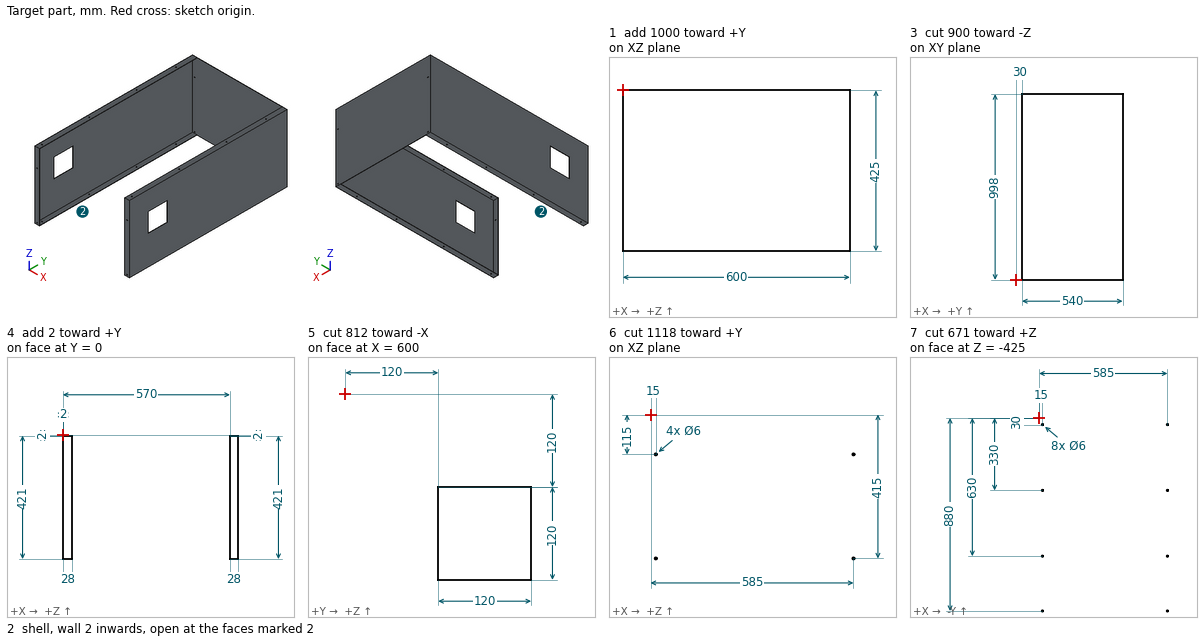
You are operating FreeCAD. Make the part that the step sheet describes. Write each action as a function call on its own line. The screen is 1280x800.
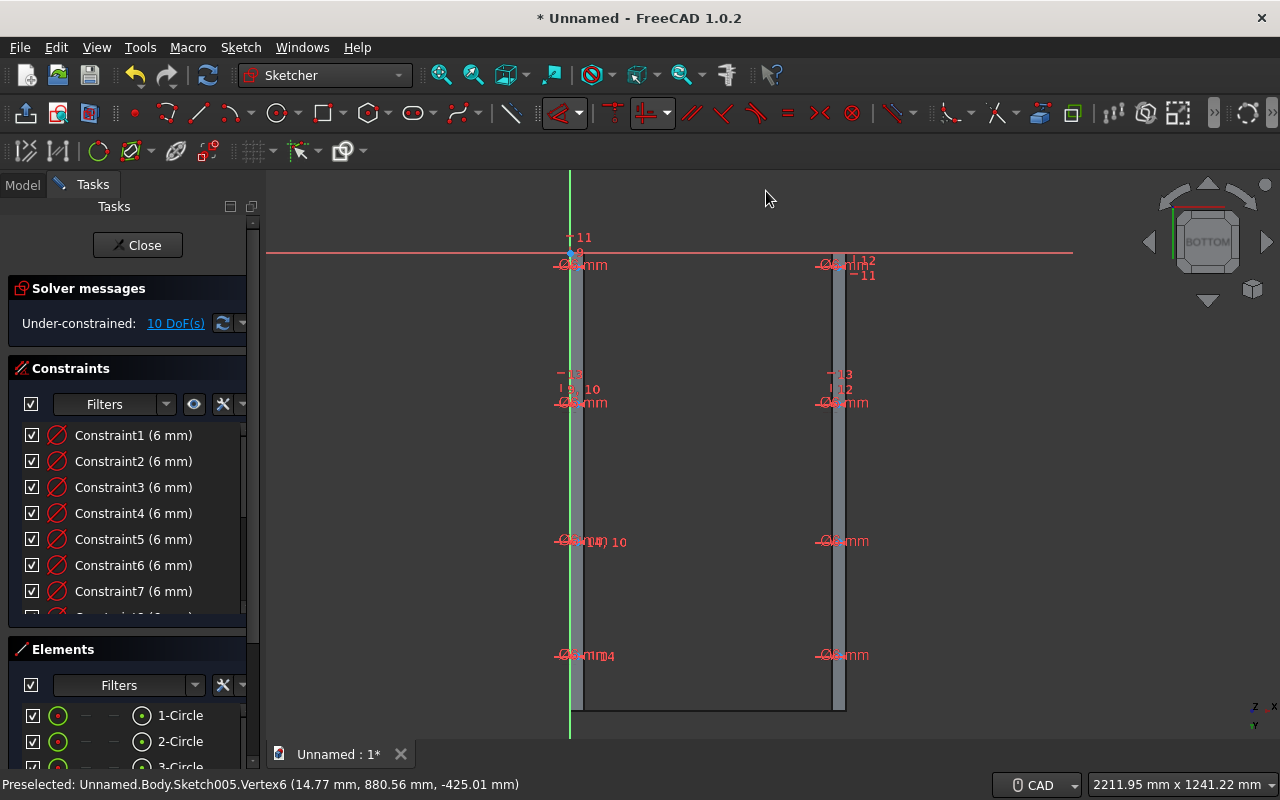
click(838, 405)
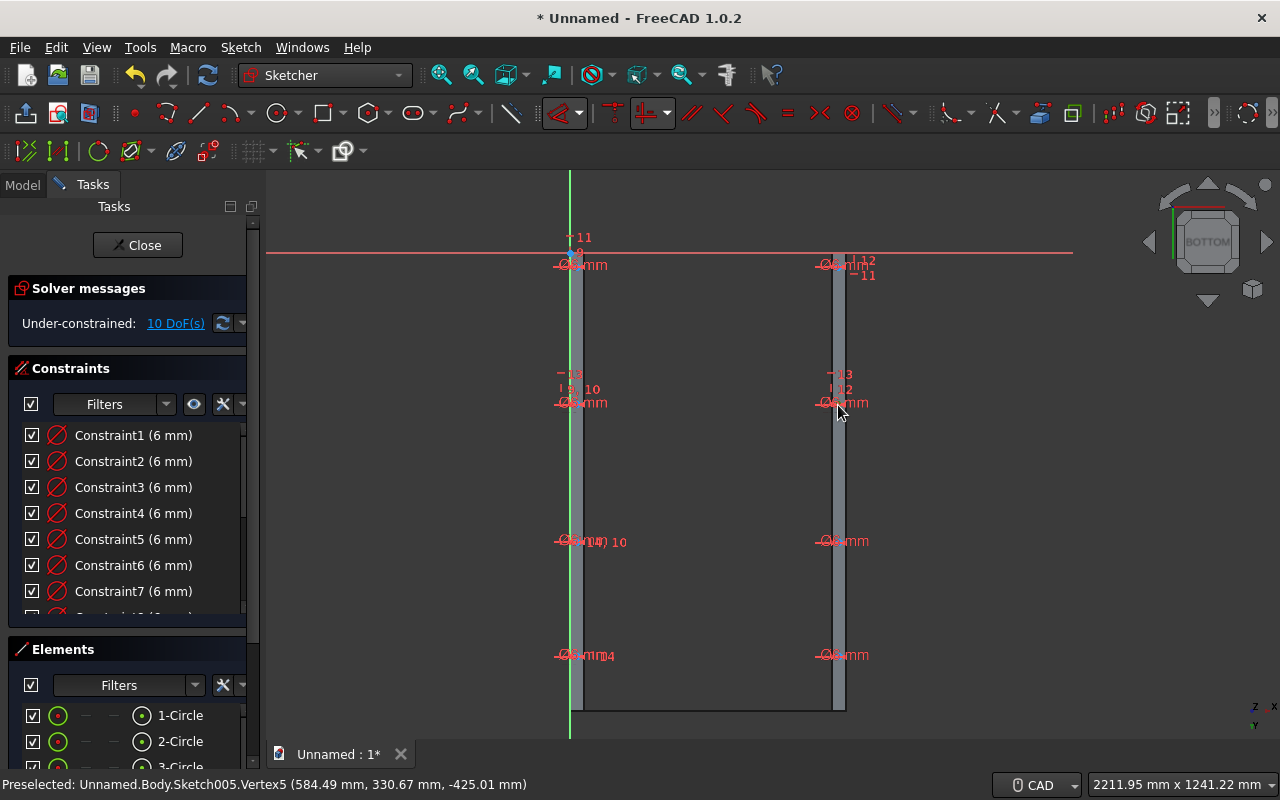
click(839, 543)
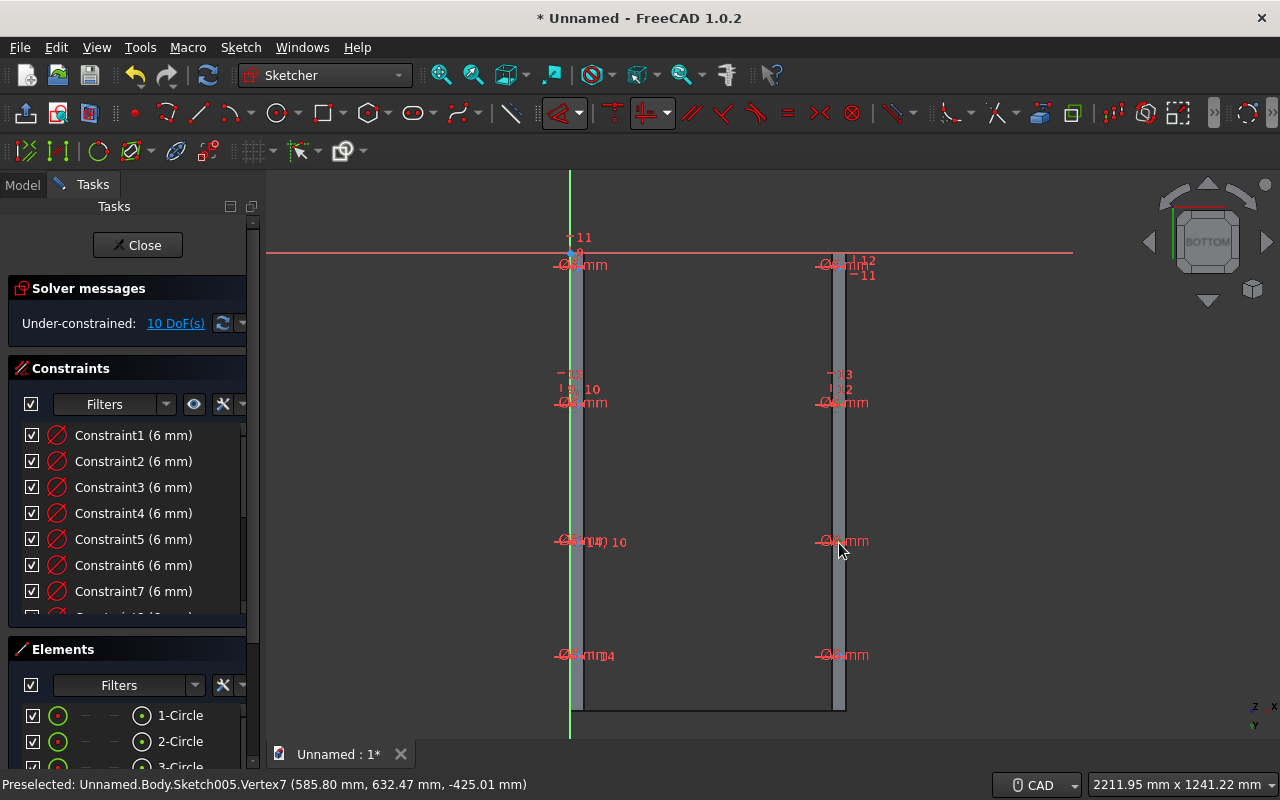
key(v)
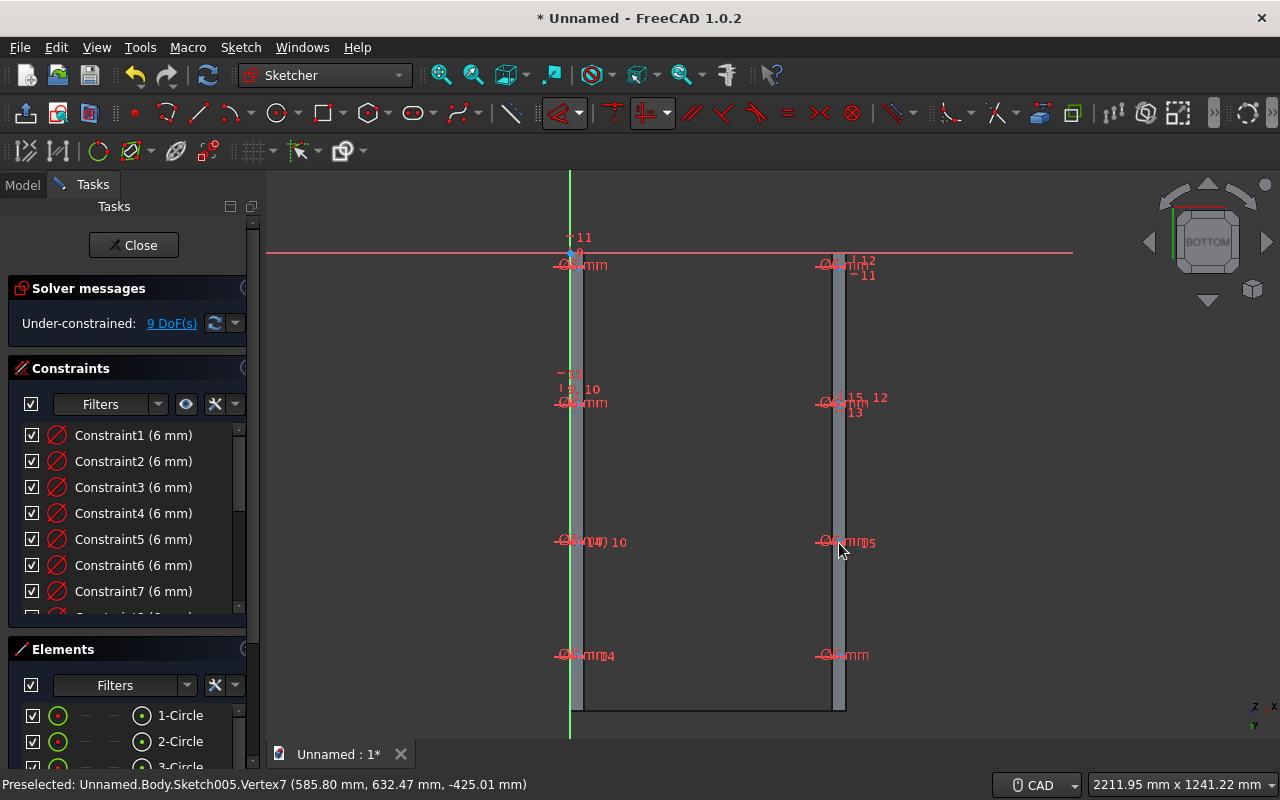
click(577, 542)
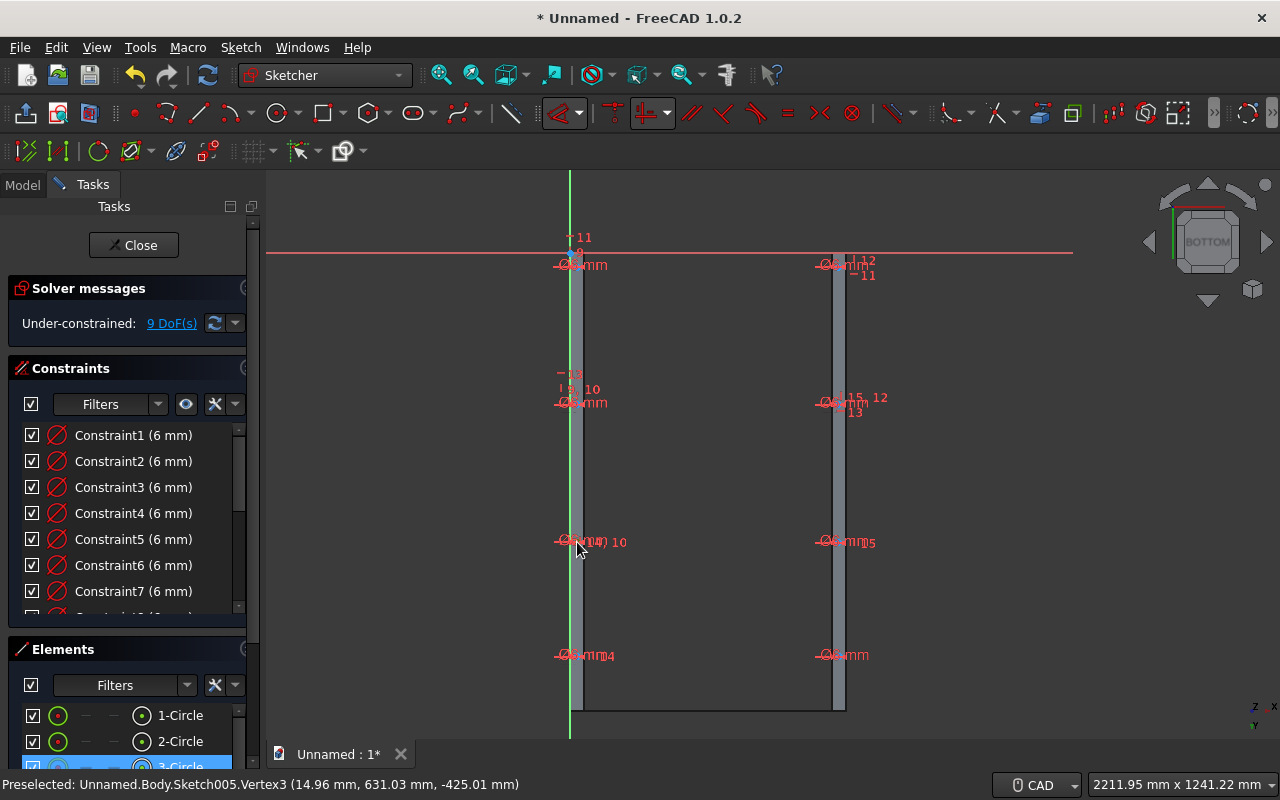
click(838, 543)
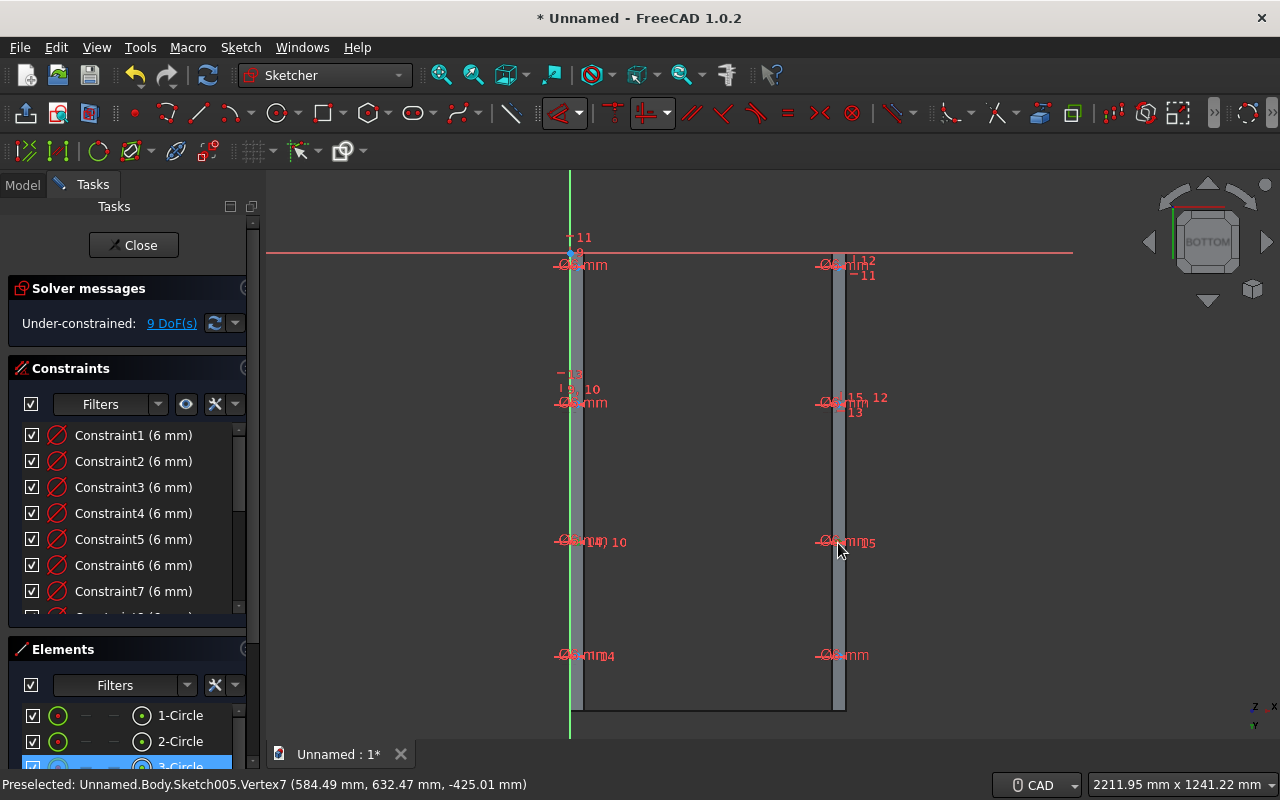
click(670, 114)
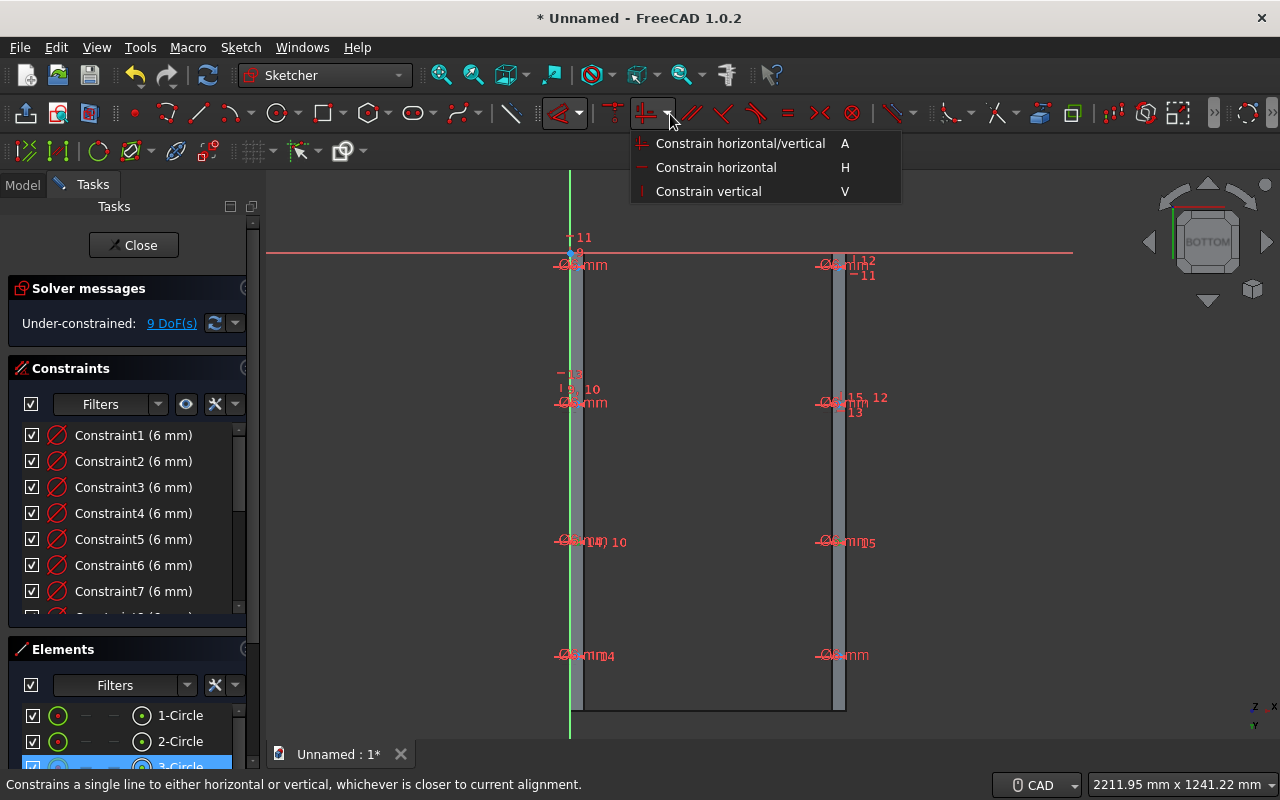
click(766, 167)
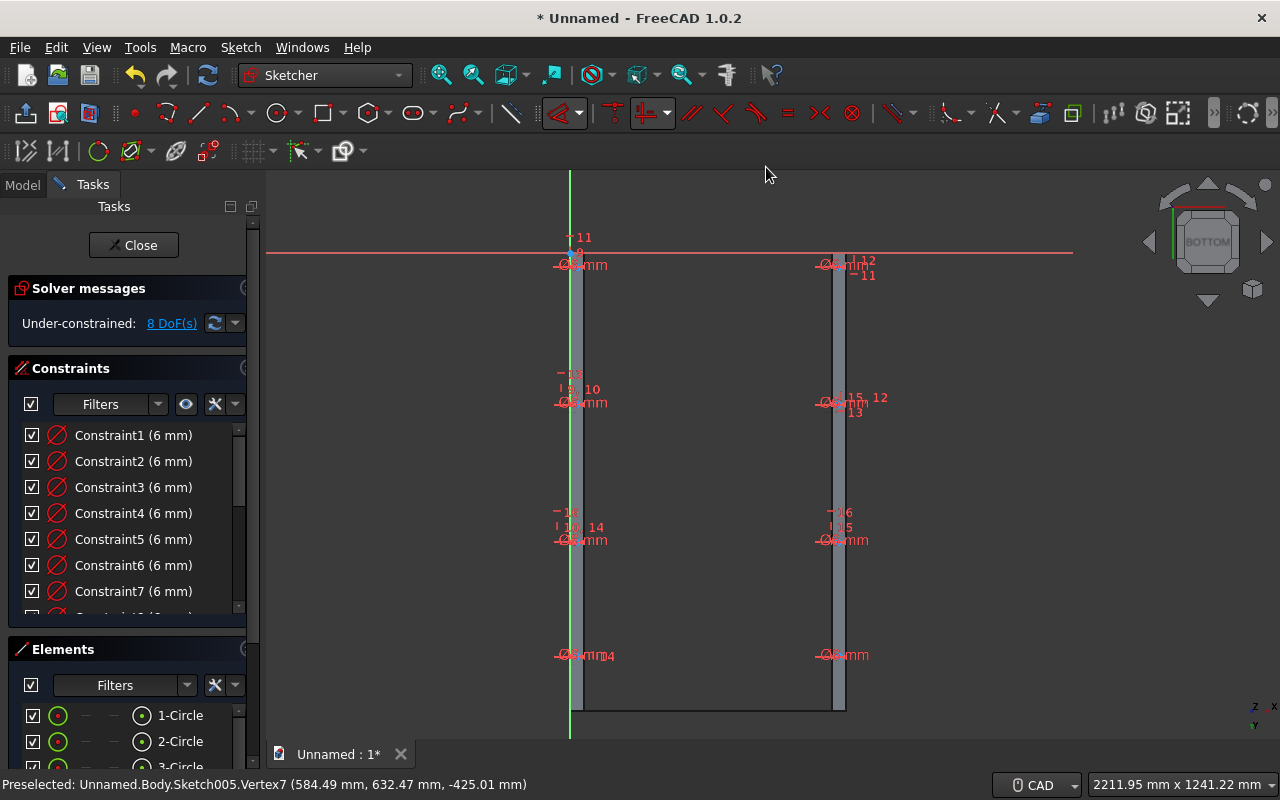
click(838, 542)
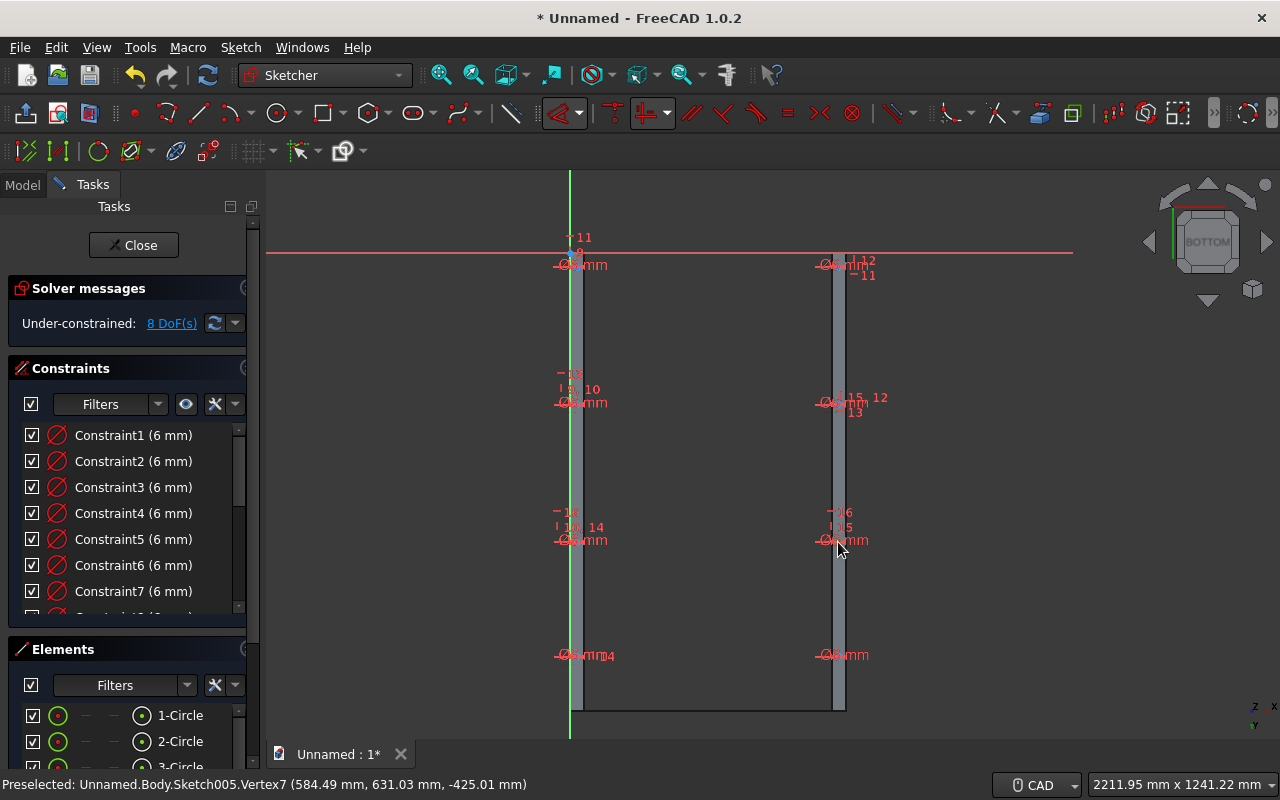
click(839, 657)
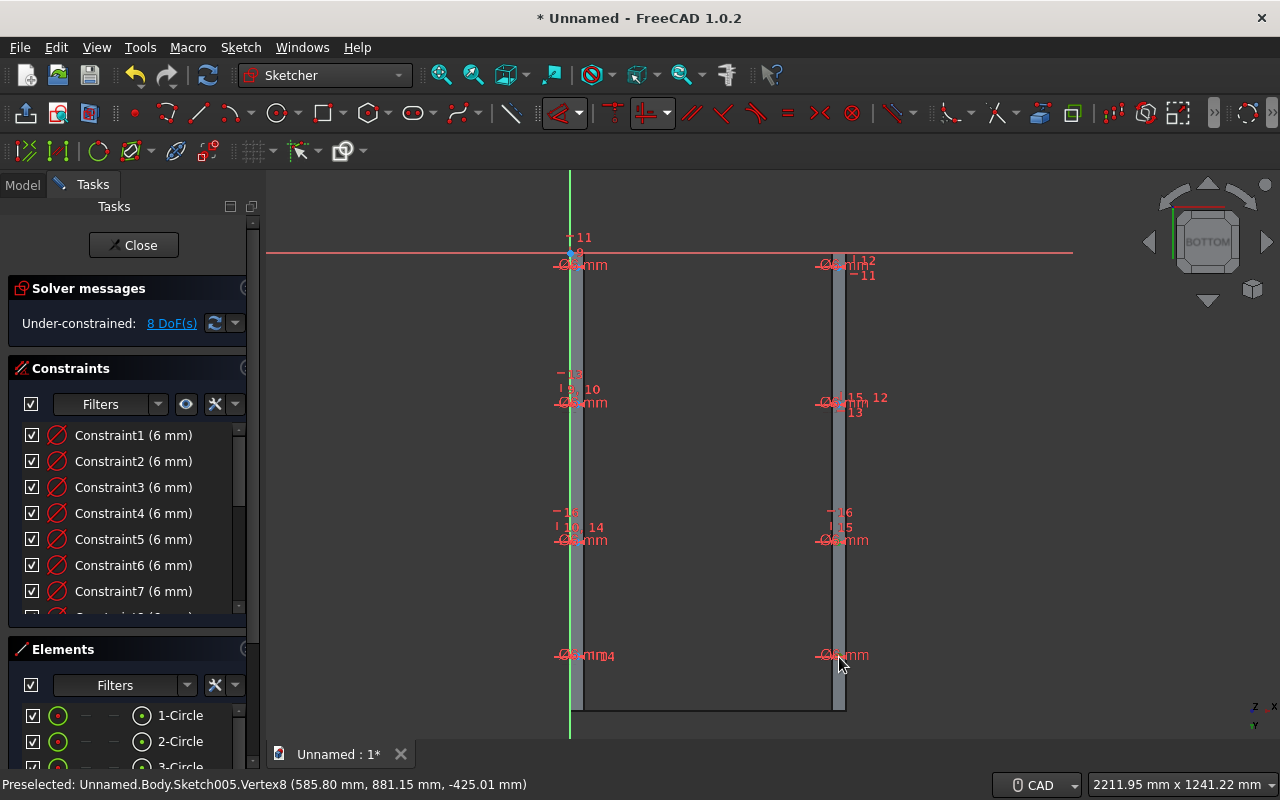
click(670, 114)